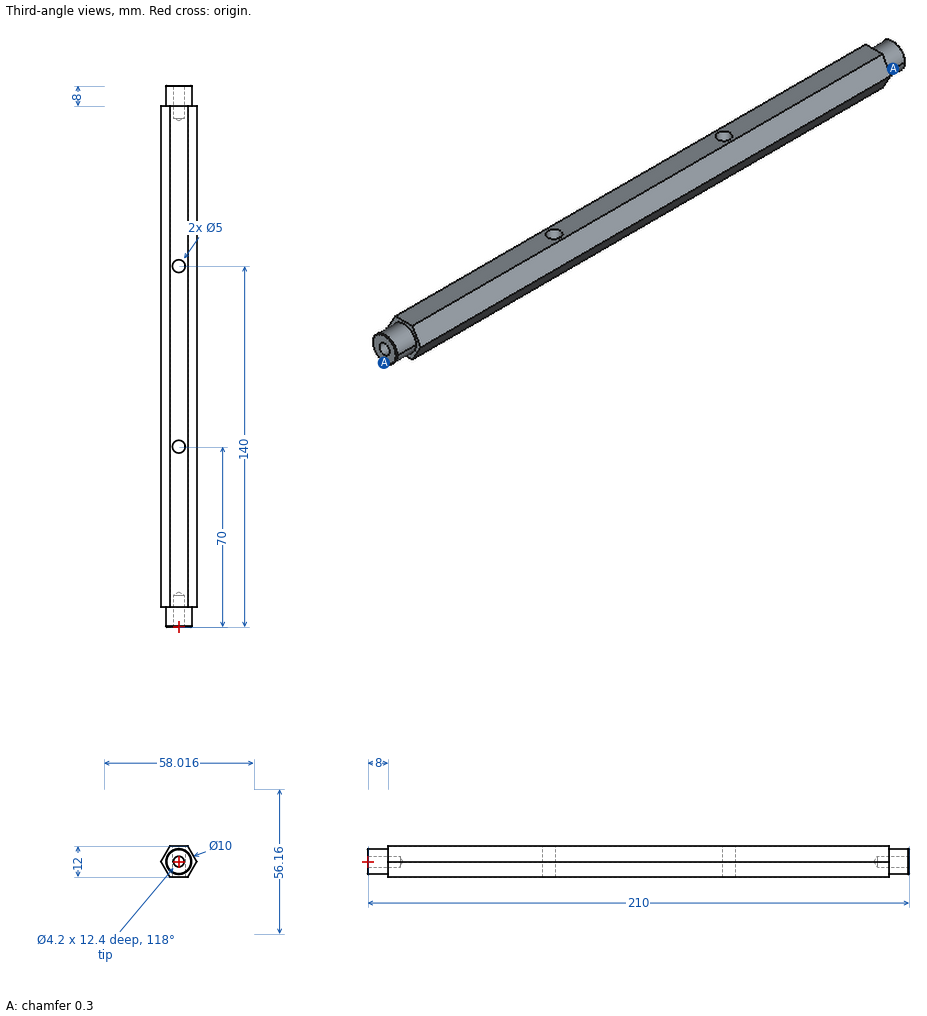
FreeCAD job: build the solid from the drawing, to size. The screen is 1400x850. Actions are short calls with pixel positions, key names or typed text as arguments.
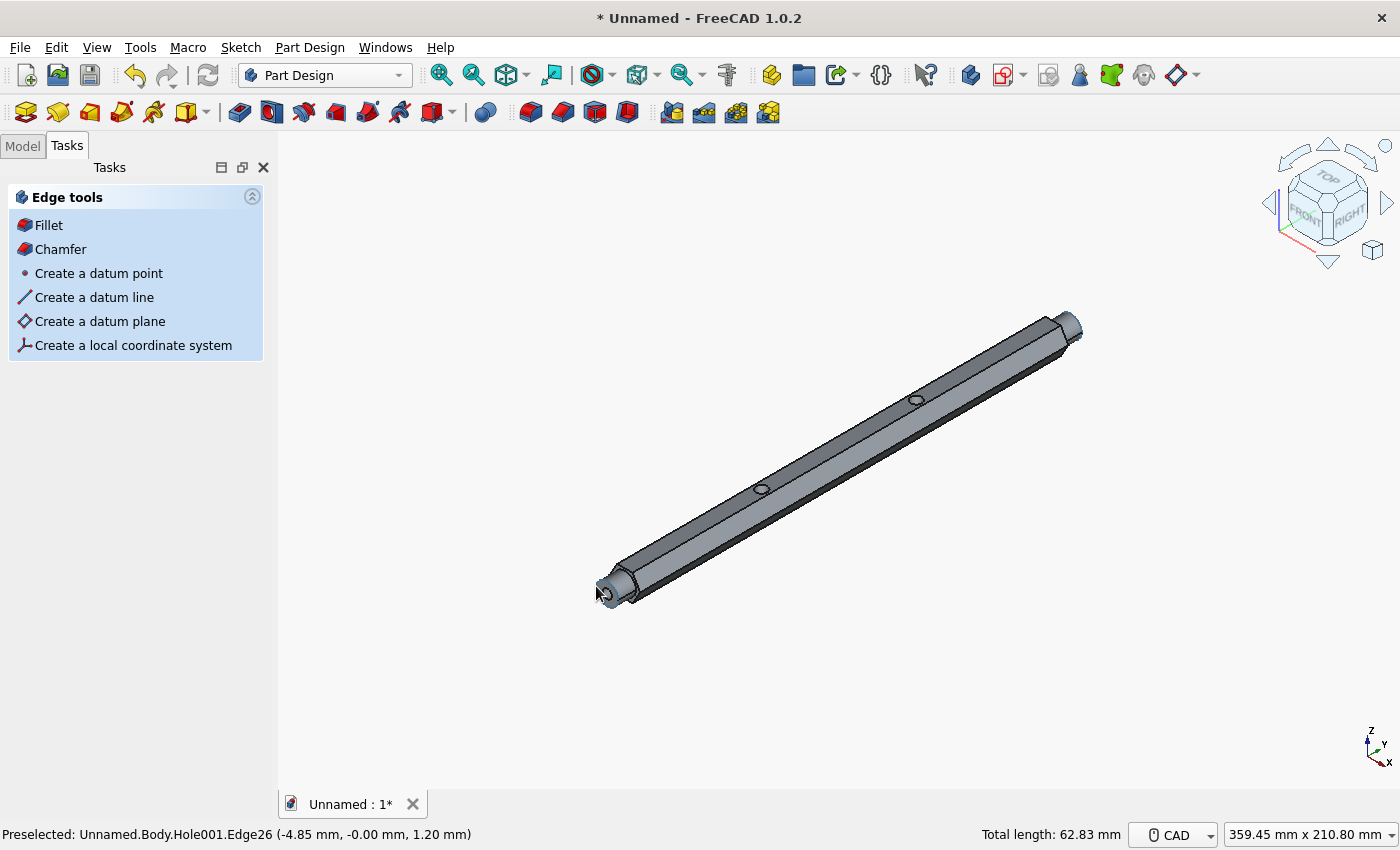
click(564, 112)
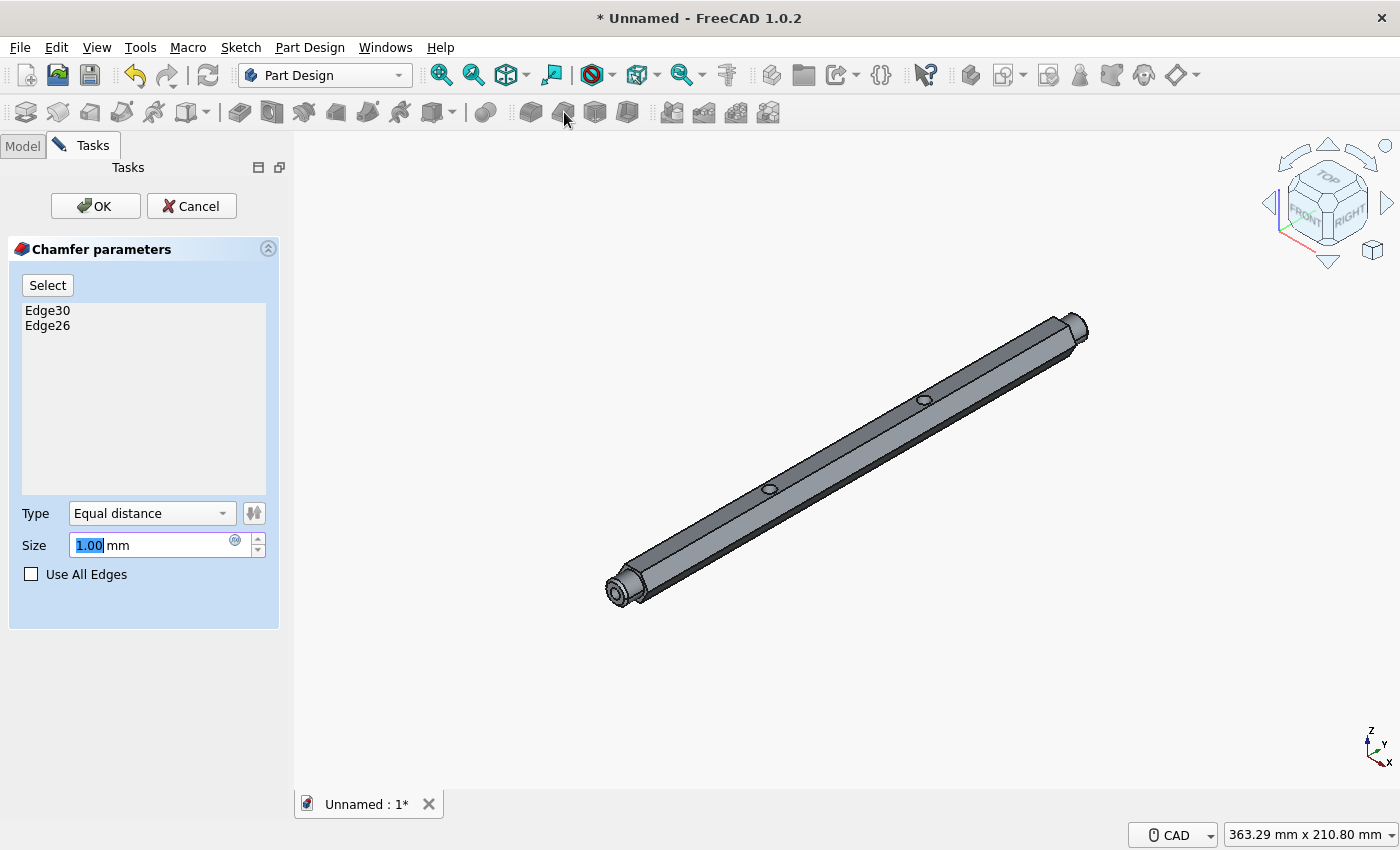
text(0.3)
key(Tab)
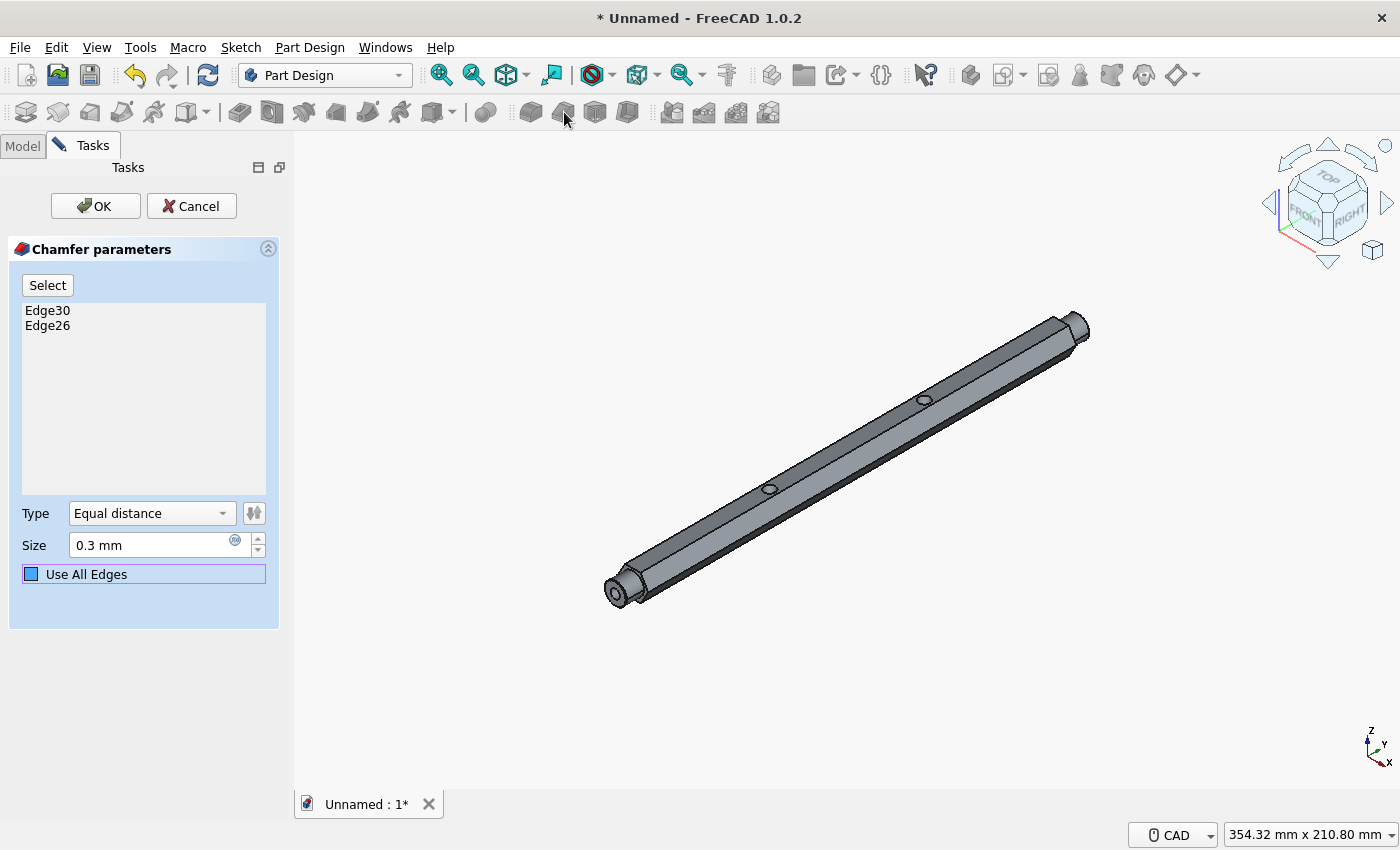
click(96, 206)